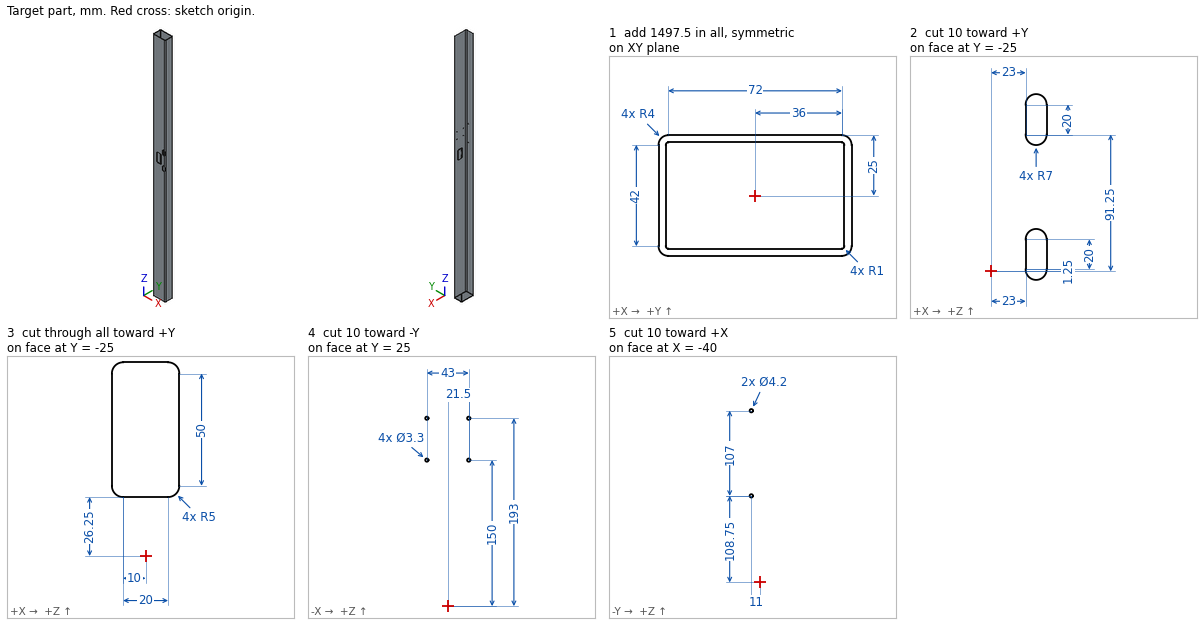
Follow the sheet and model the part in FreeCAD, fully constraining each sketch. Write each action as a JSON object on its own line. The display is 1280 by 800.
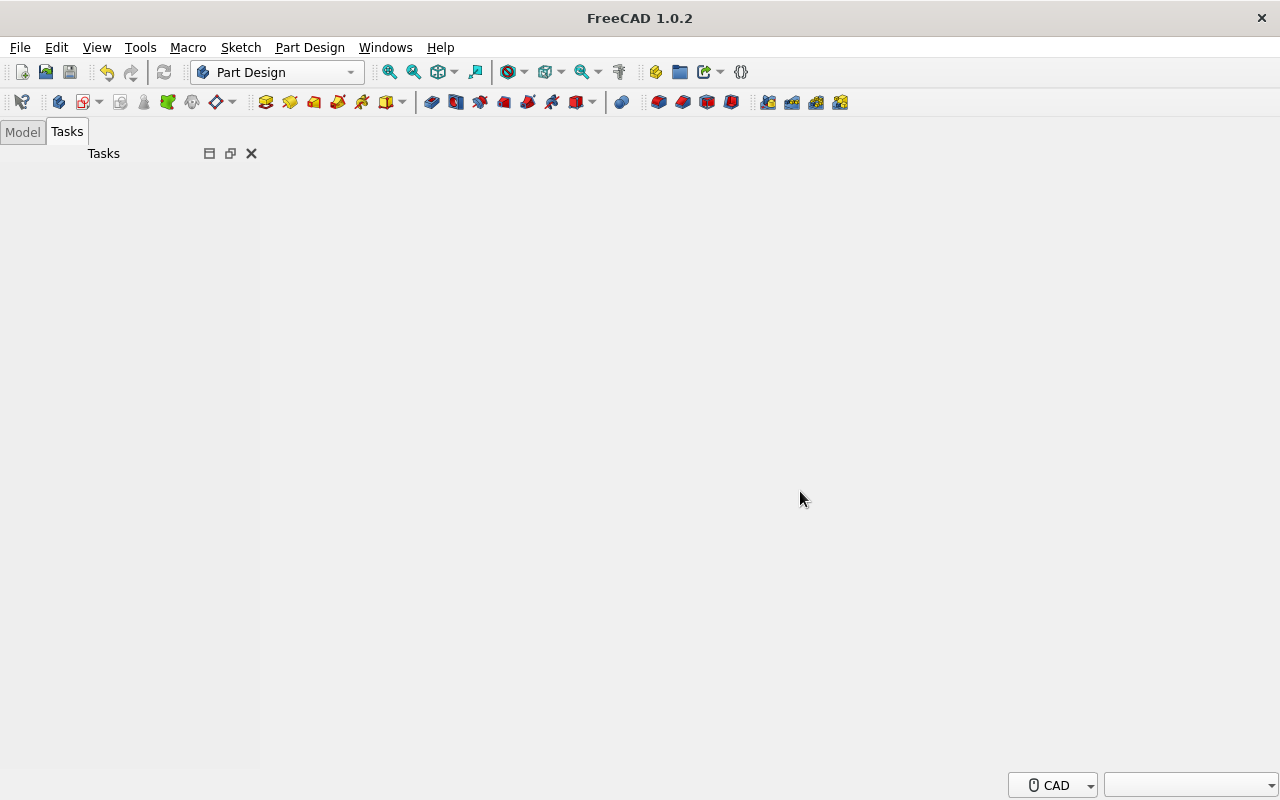
{"action": "key", "text": "ctrl+n"}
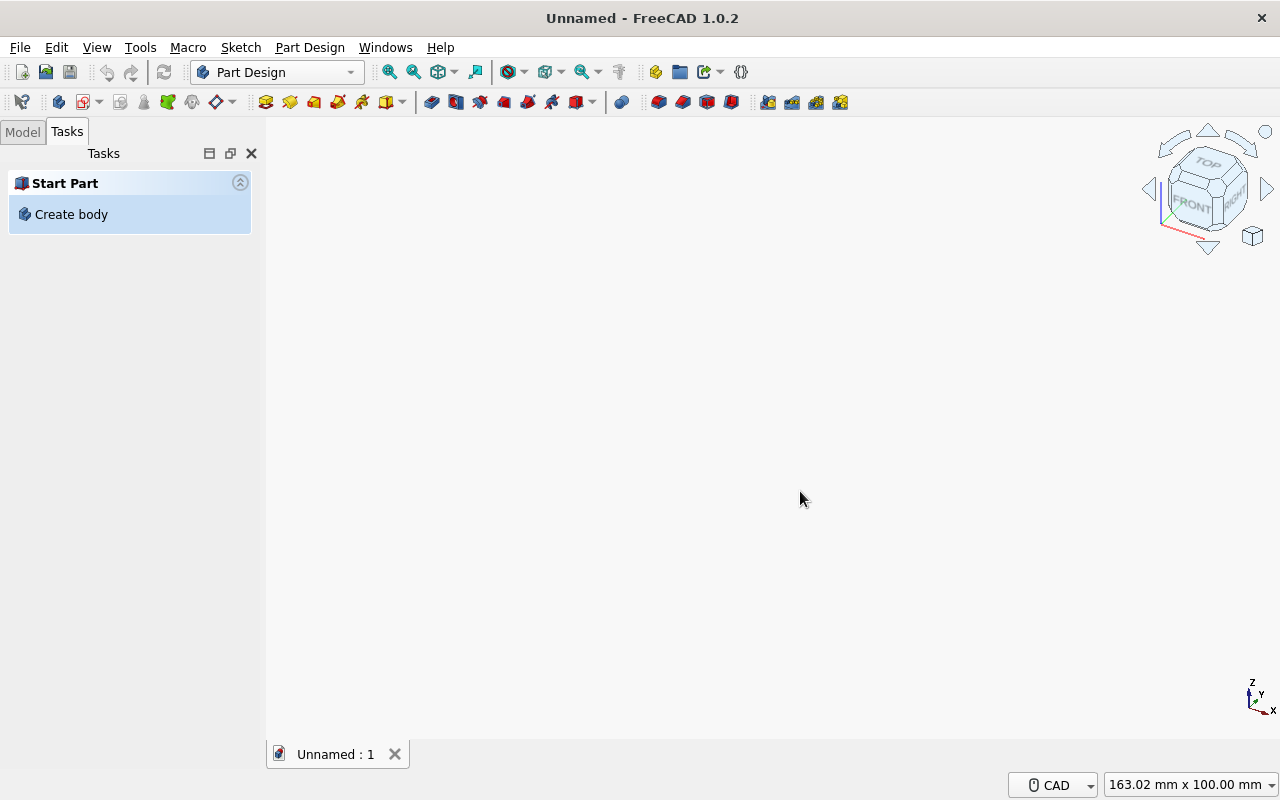
{"action": "left_click", "coordinate": [84, 102]}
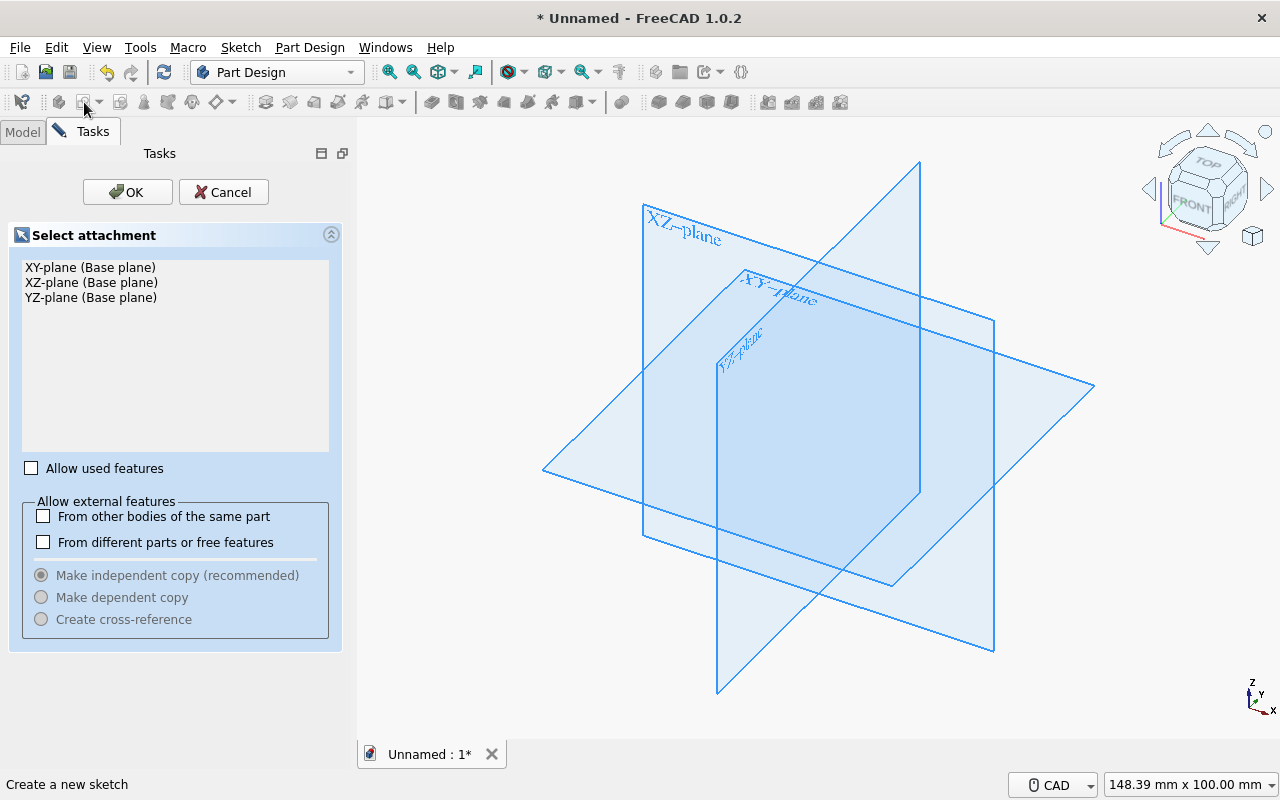
{"action": "left_click", "coordinate": [82, 268]}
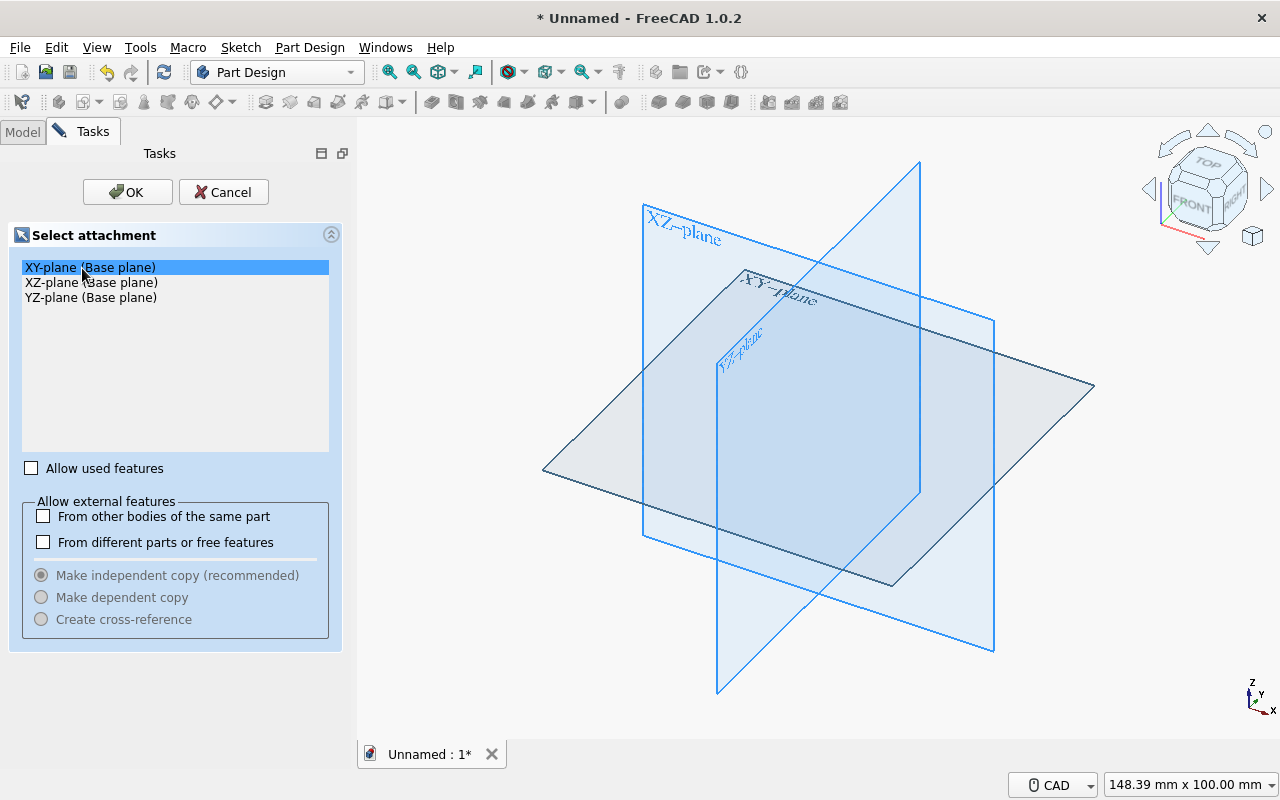
{"action": "left_click", "coordinate": [128, 192]}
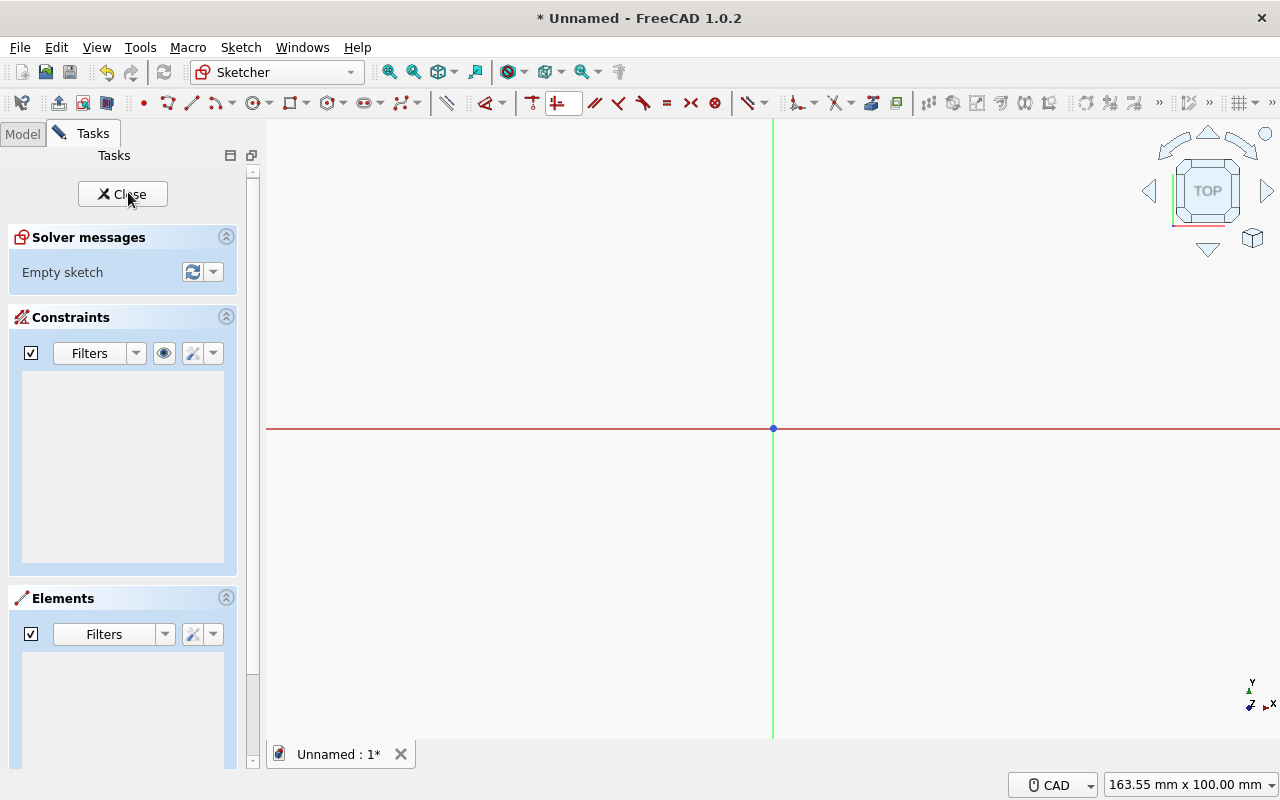
{"action": "key", "text": "g l"}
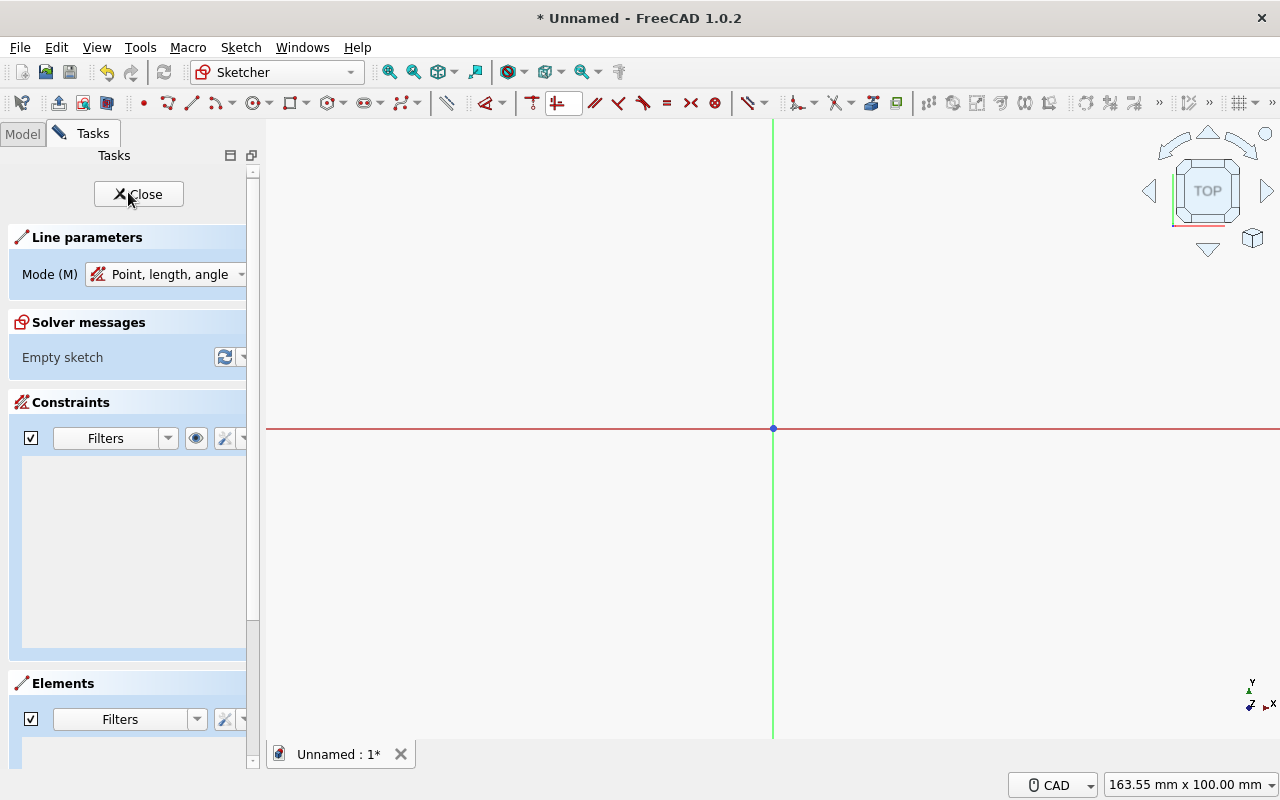
{"action": "left_click", "coordinate": [996, 274]}
{"action": "left_click", "coordinate": [550, 274]}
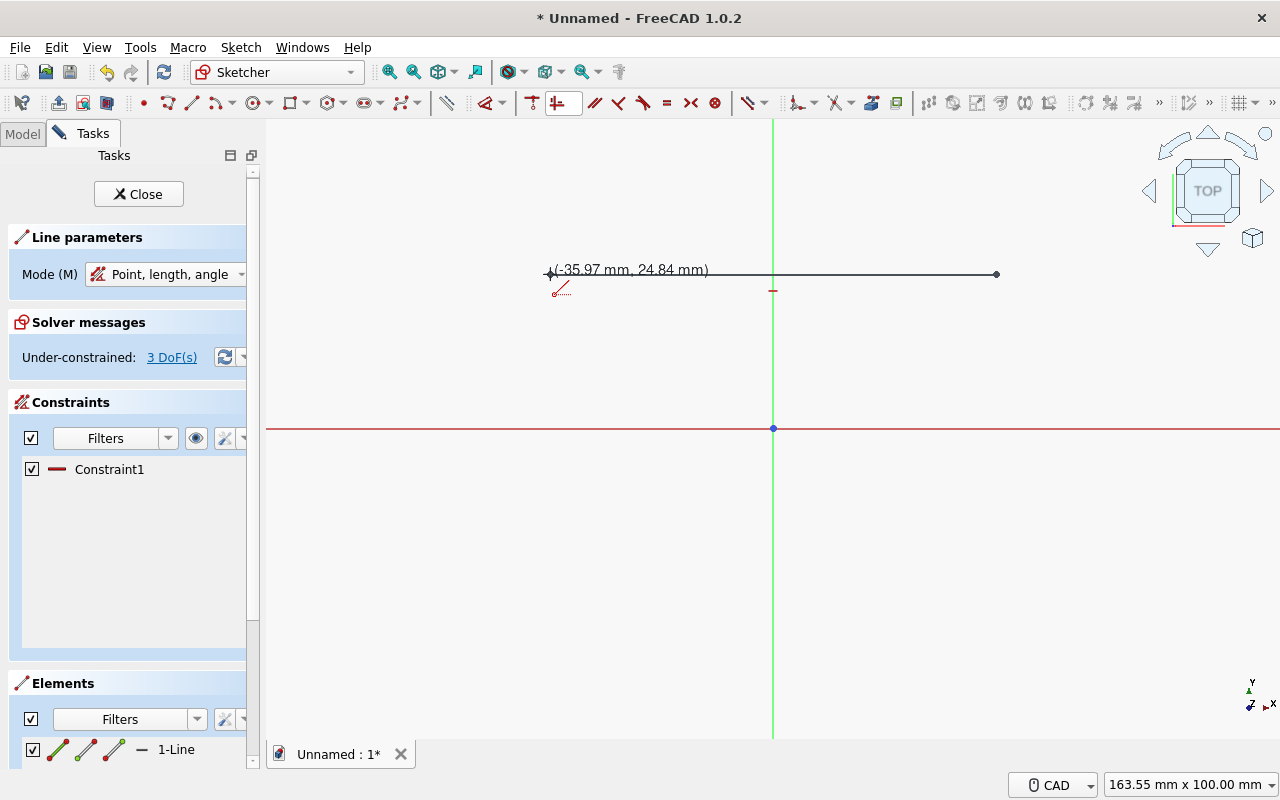
{"action": "left_click", "coordinate": [525, 299]}
{"action": "left_click", "coordinate": [525, 559]}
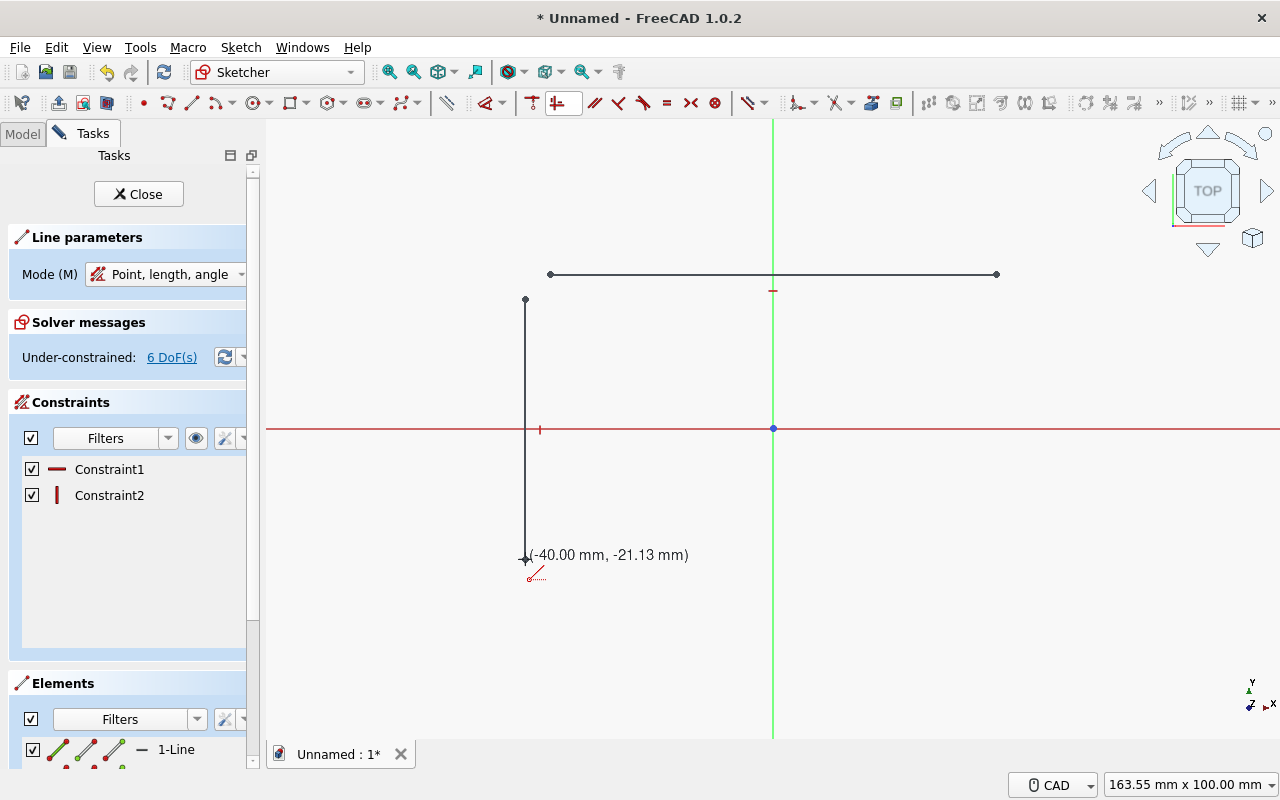
{"action": "left_click", "coordinate": [550, 584]}
{"action": "left_click", "coordinate": [996, 584]}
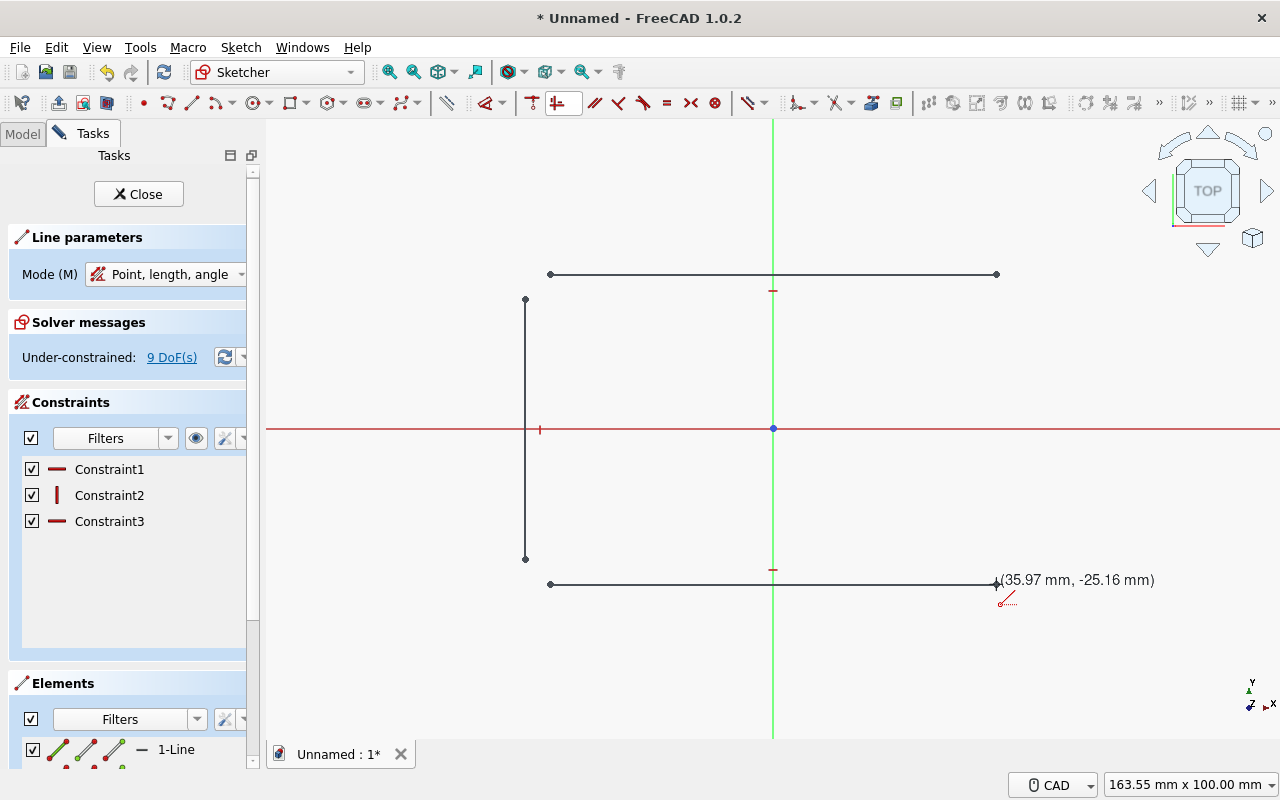
{"action": "left_click", "coordinate": [1021, 559]}
{"action": "left_click", "coordinate": [1021, 299]}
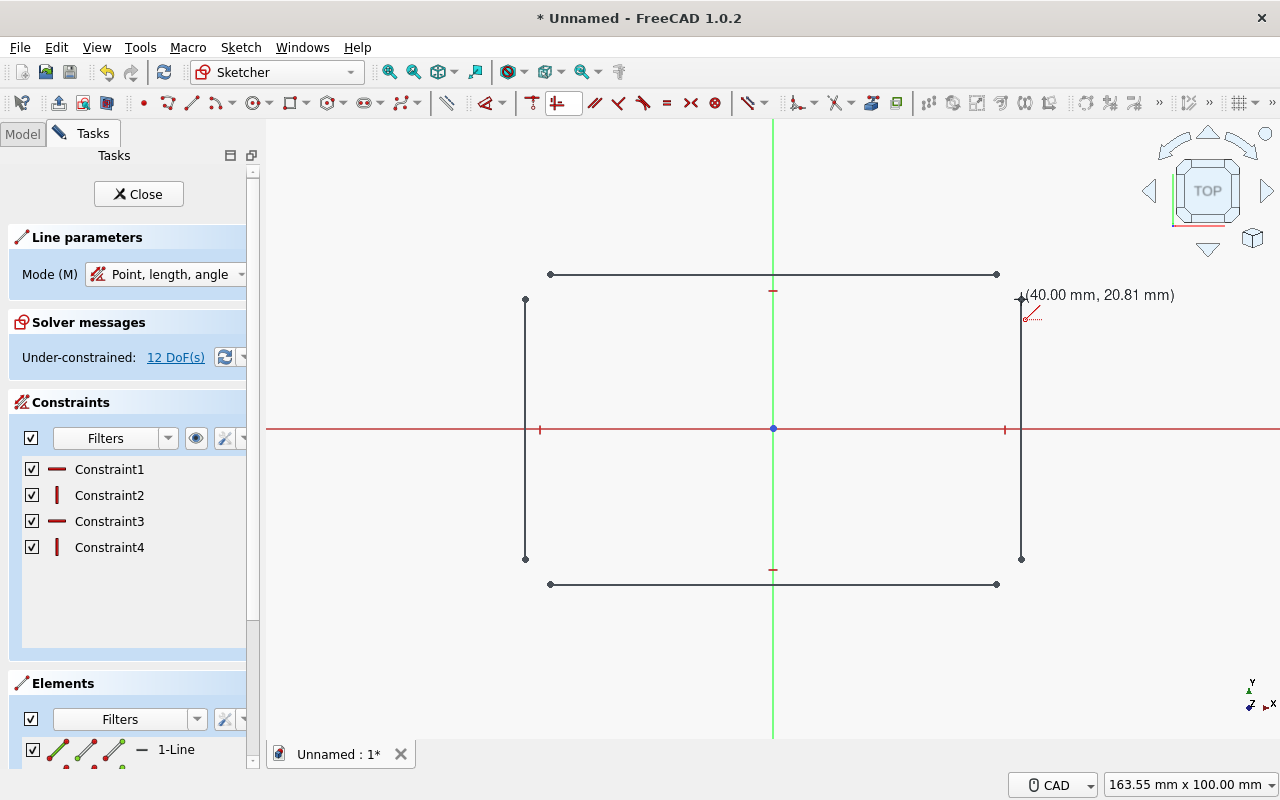
{"action": "key", "text": "g 3 a"}